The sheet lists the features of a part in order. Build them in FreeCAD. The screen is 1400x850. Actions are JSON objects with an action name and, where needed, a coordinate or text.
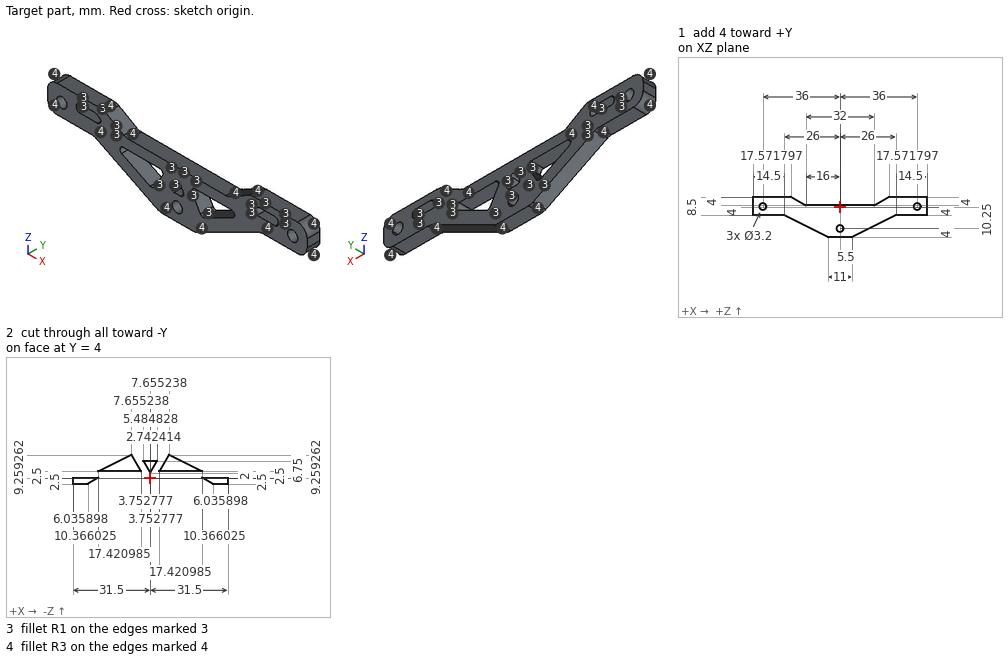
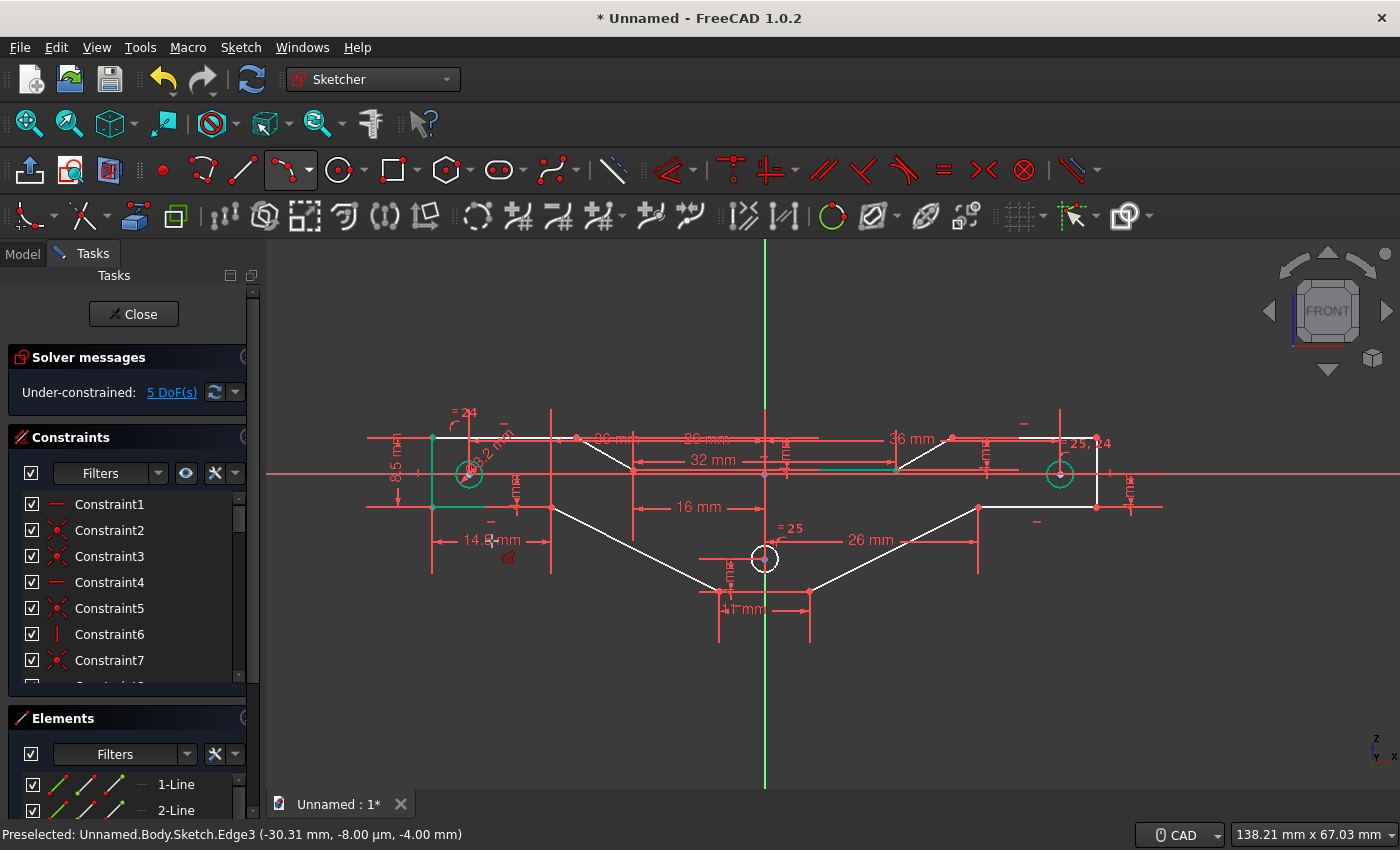
{"action": "left_click", "coordinate": [1061, 507]}
{"action": "left_click", "coordinate": [1037, 541]}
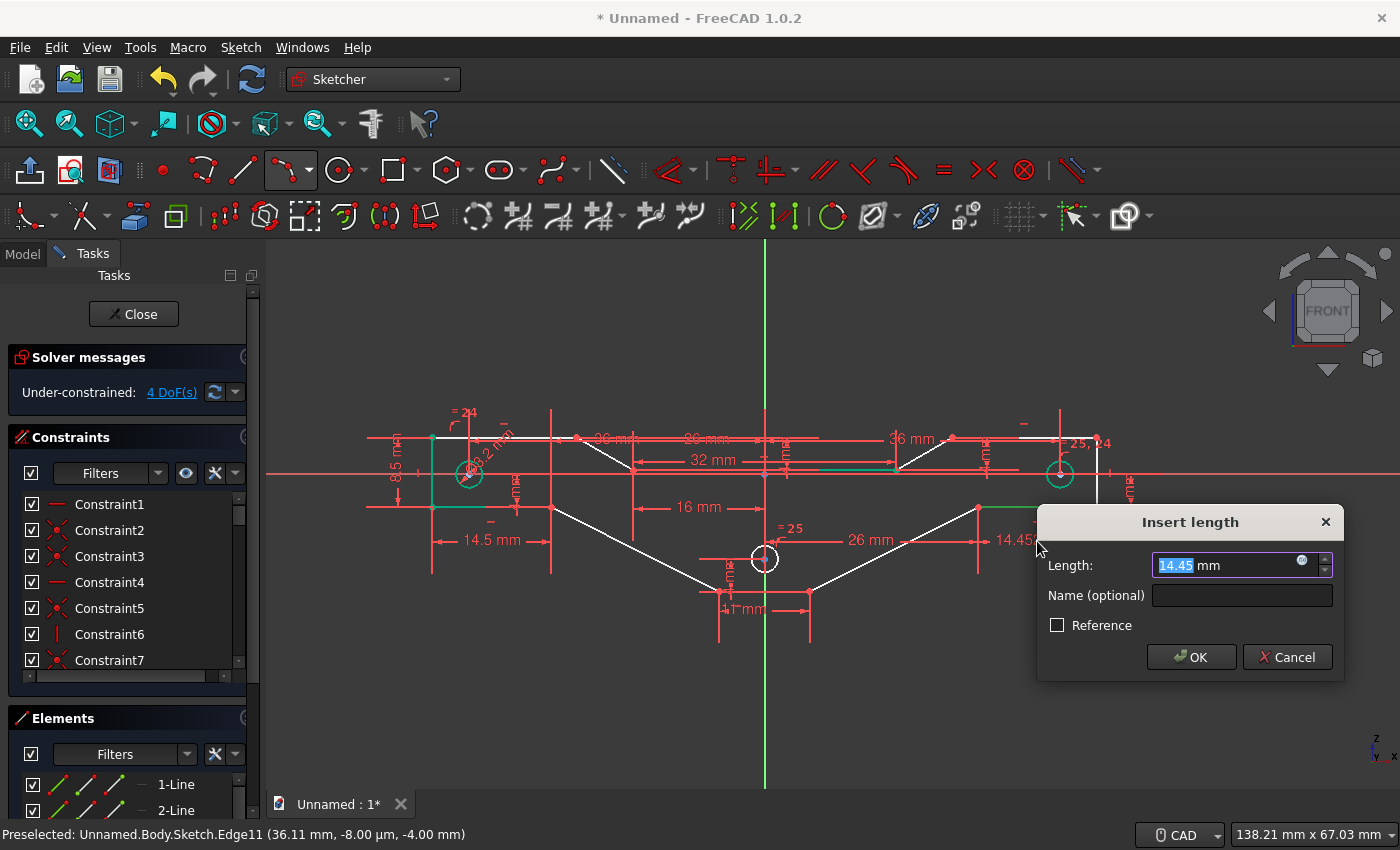
{"action": "type", "text": "14.5"}
{"action": "key", "text": "Return"}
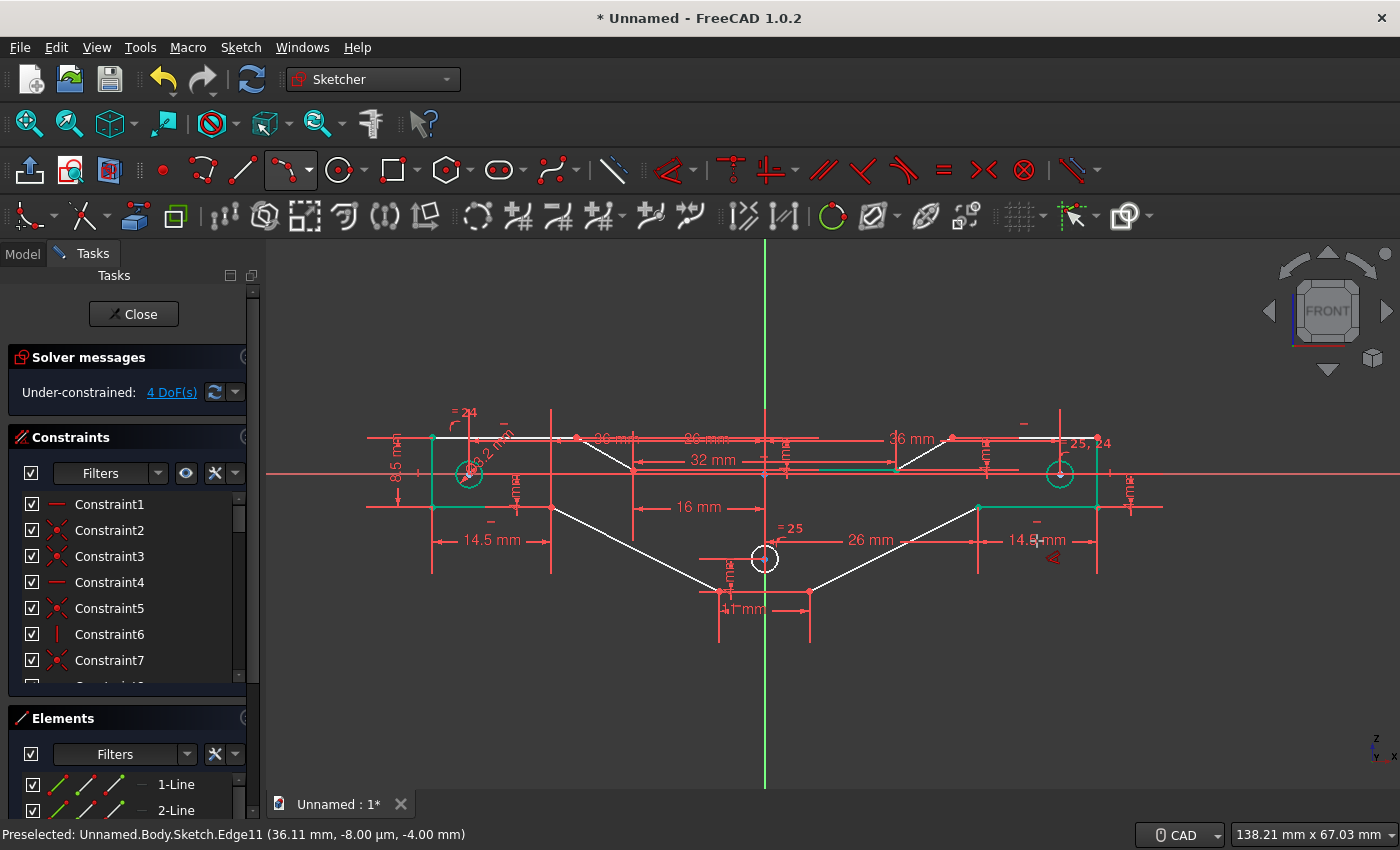
{"action": "left_click", "coordinate": [810, 592]}
{"action": "left_click", "coordinate": [787, 650]}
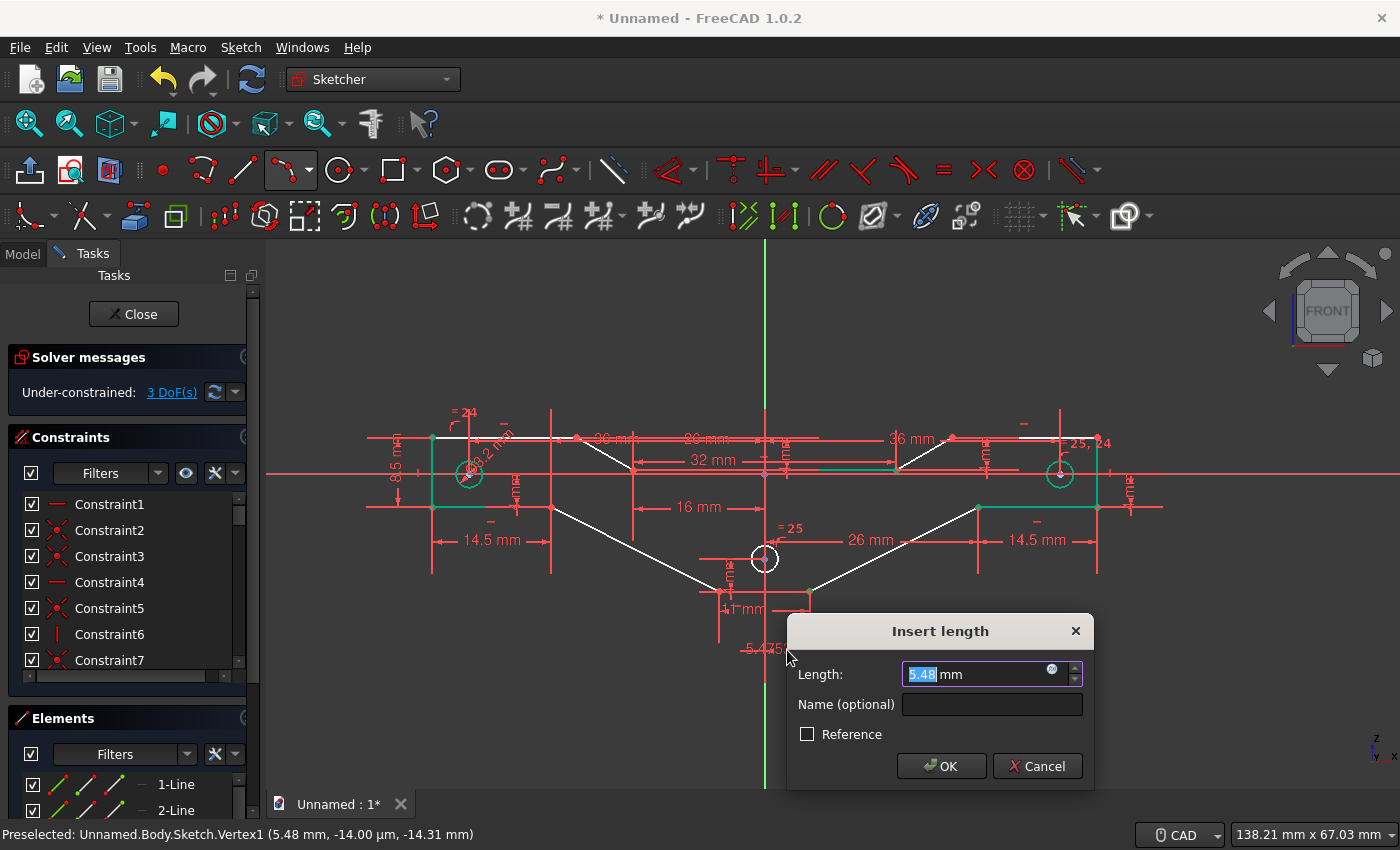
{"action": "type", "text": "5.5"}
{"action": "key", "text": "Return"}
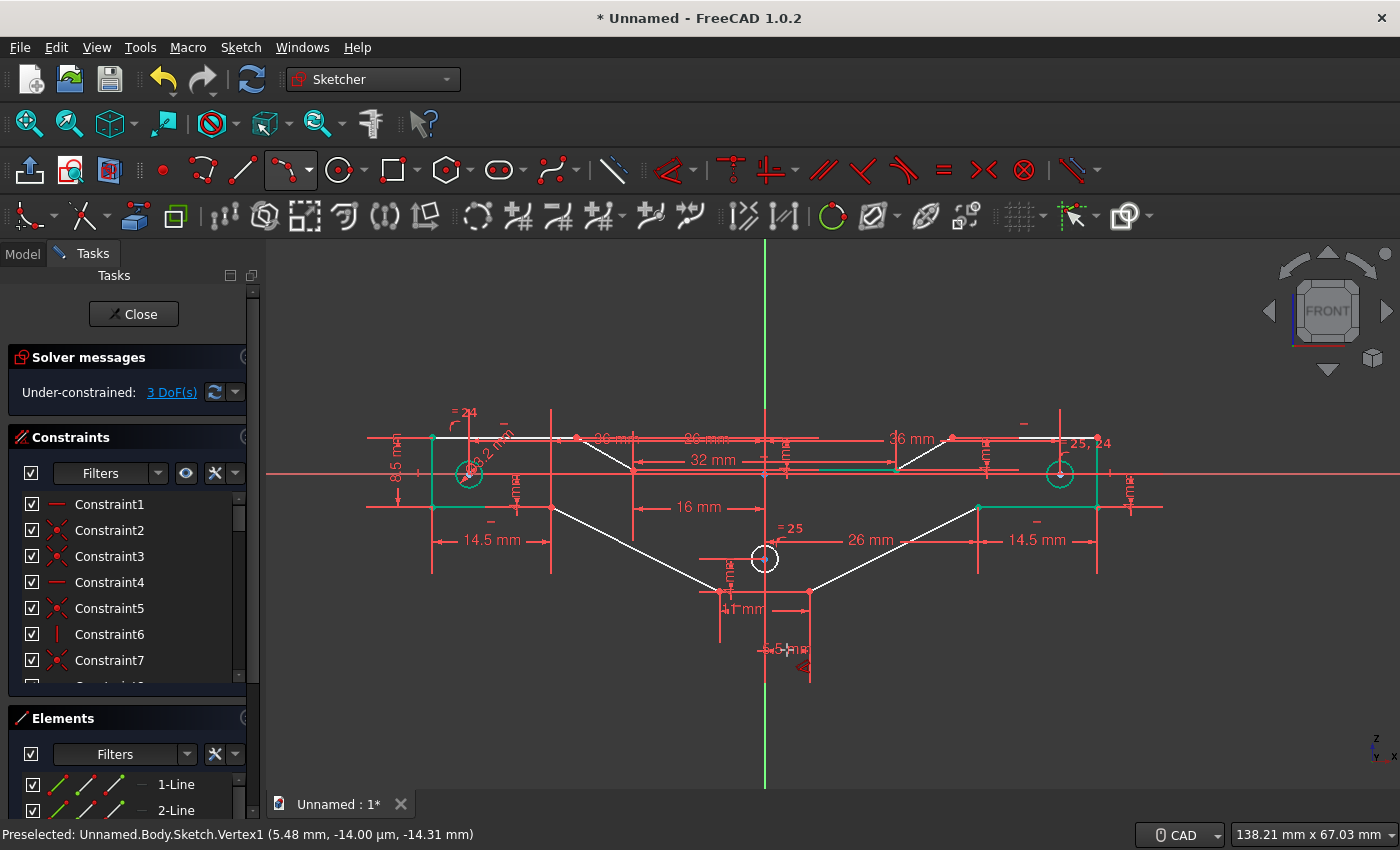
{"action": "left_click", "coordinate": [765, 559]}
{"action": "left_click", "coordinate": [799, 517]}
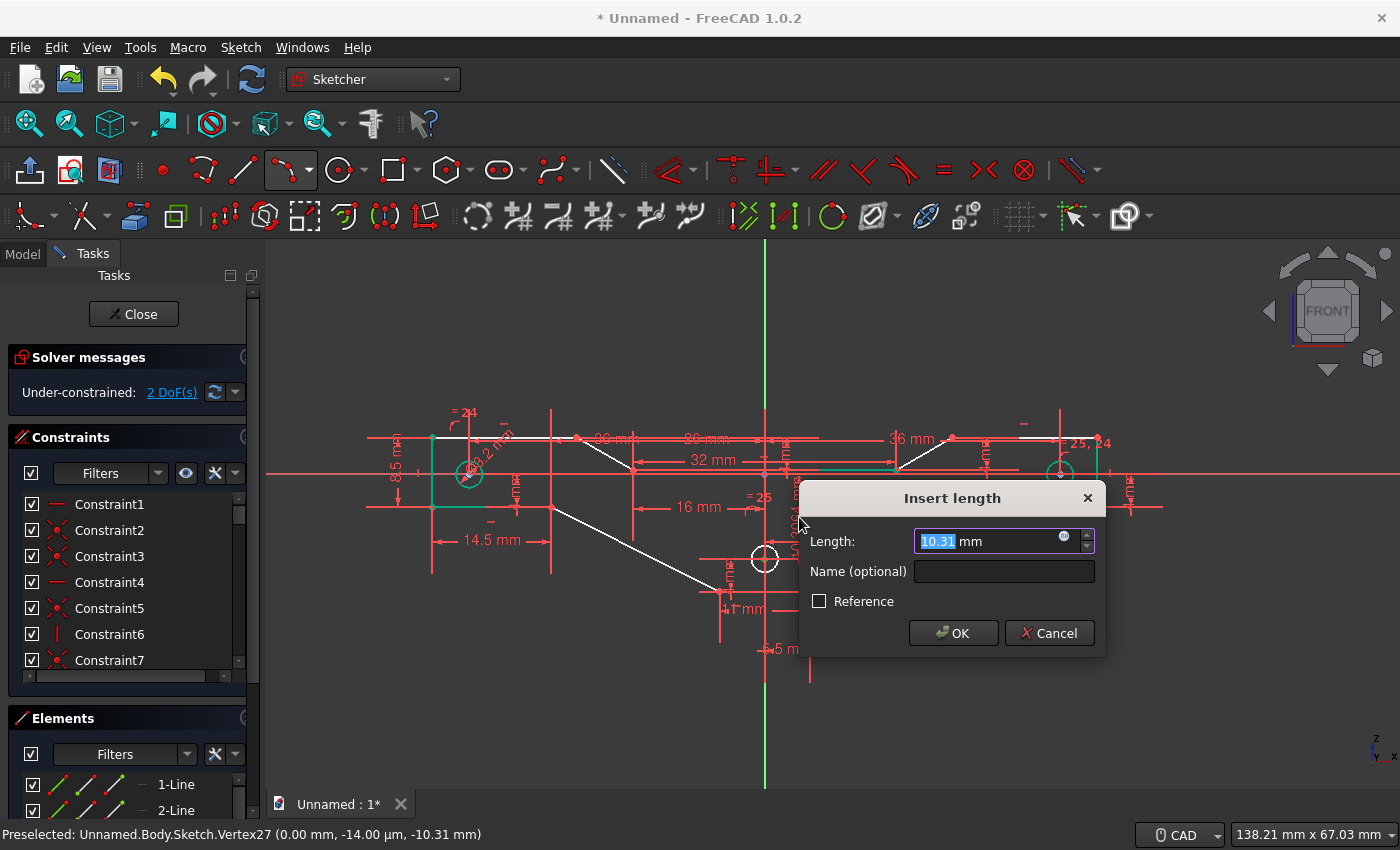
{"action": "type", "text": "10.25"}
{"action": "key", "text": "Return"}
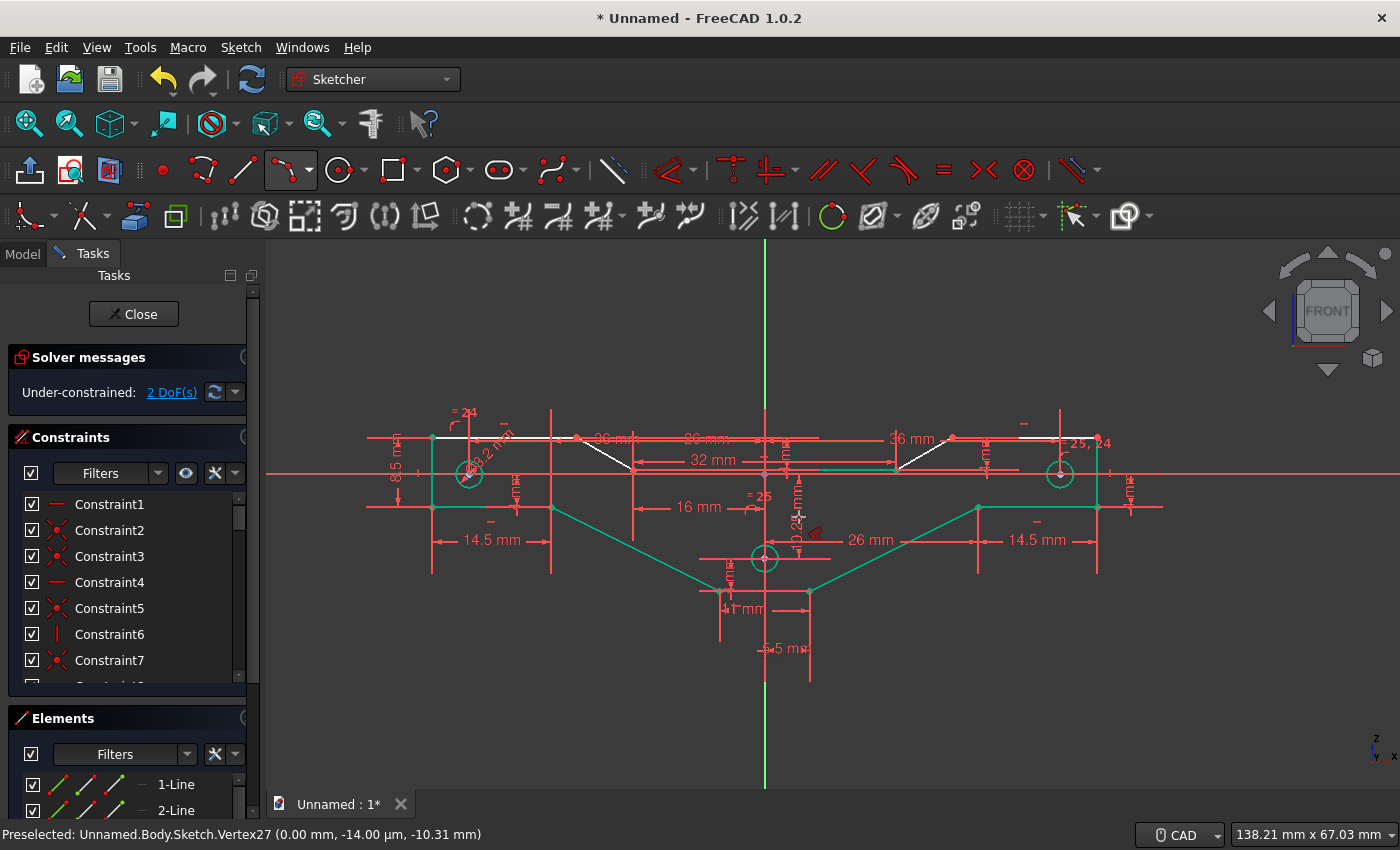
{"action": "left_click", "coordinate": [476, 438]}
{"action": "left_click", "coordinate": [504, 404]}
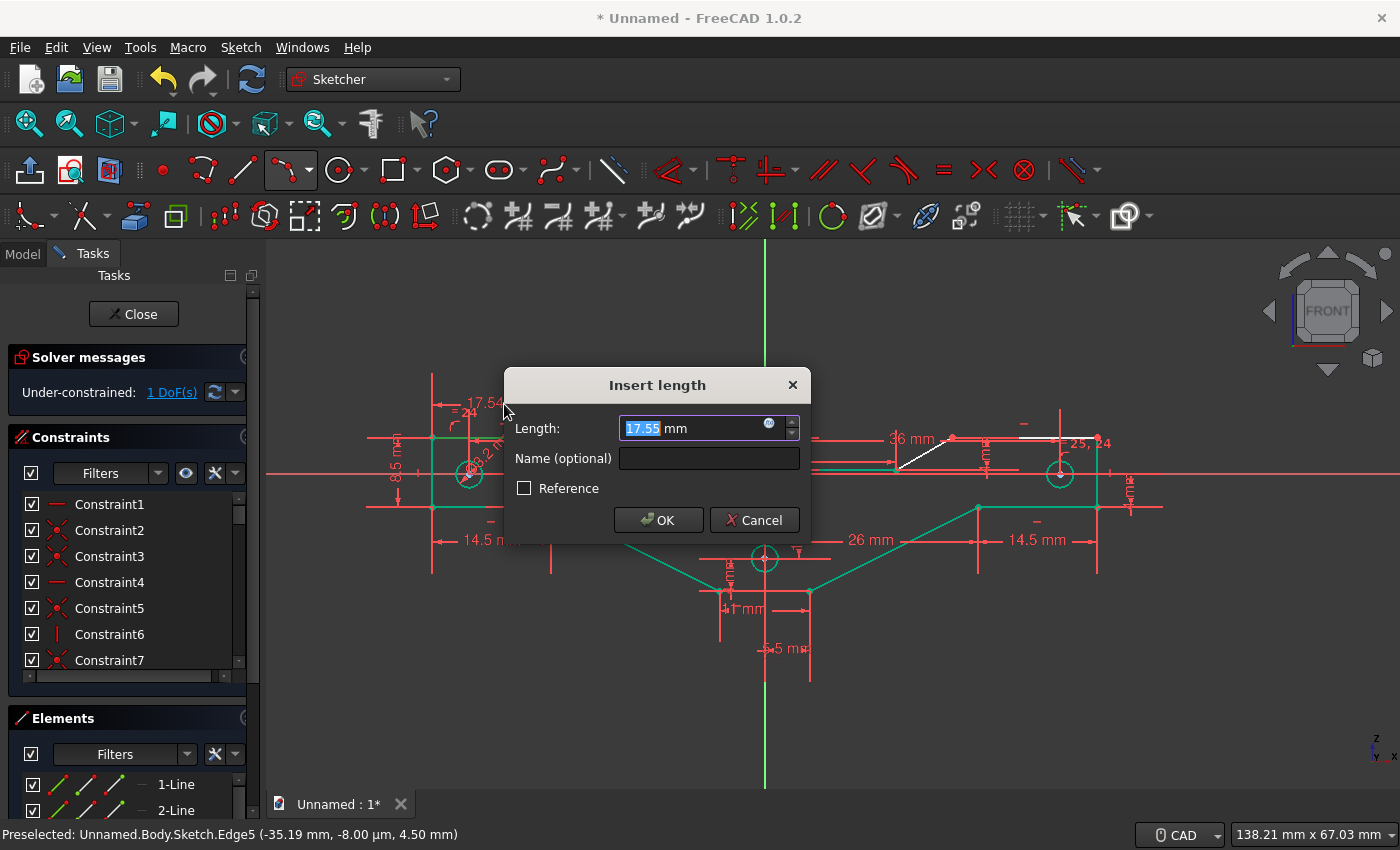
{"action": "type", "text": "17.571797"}
{"action": "key", "text": "Return"}